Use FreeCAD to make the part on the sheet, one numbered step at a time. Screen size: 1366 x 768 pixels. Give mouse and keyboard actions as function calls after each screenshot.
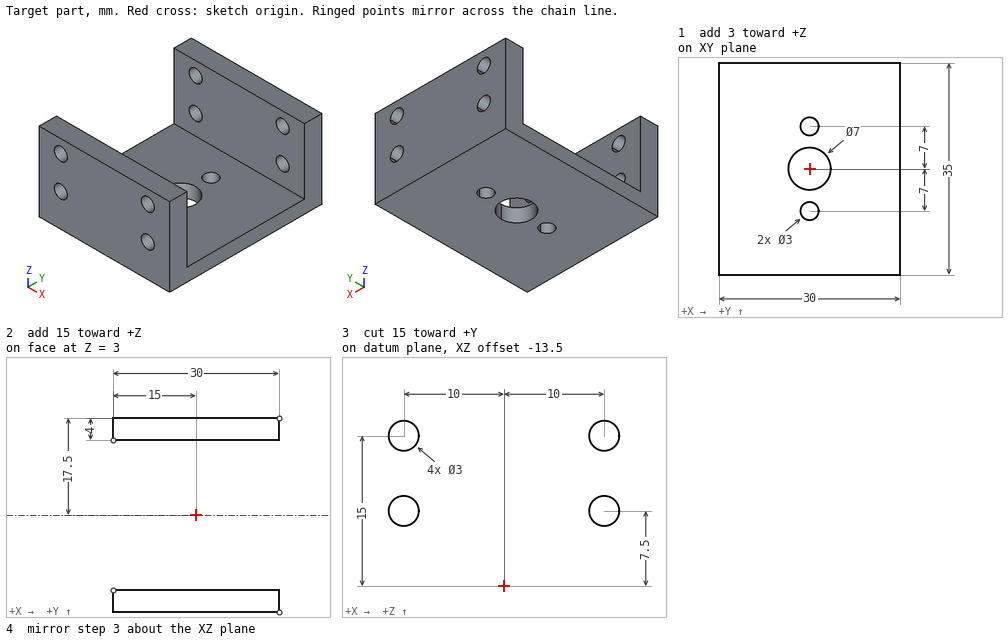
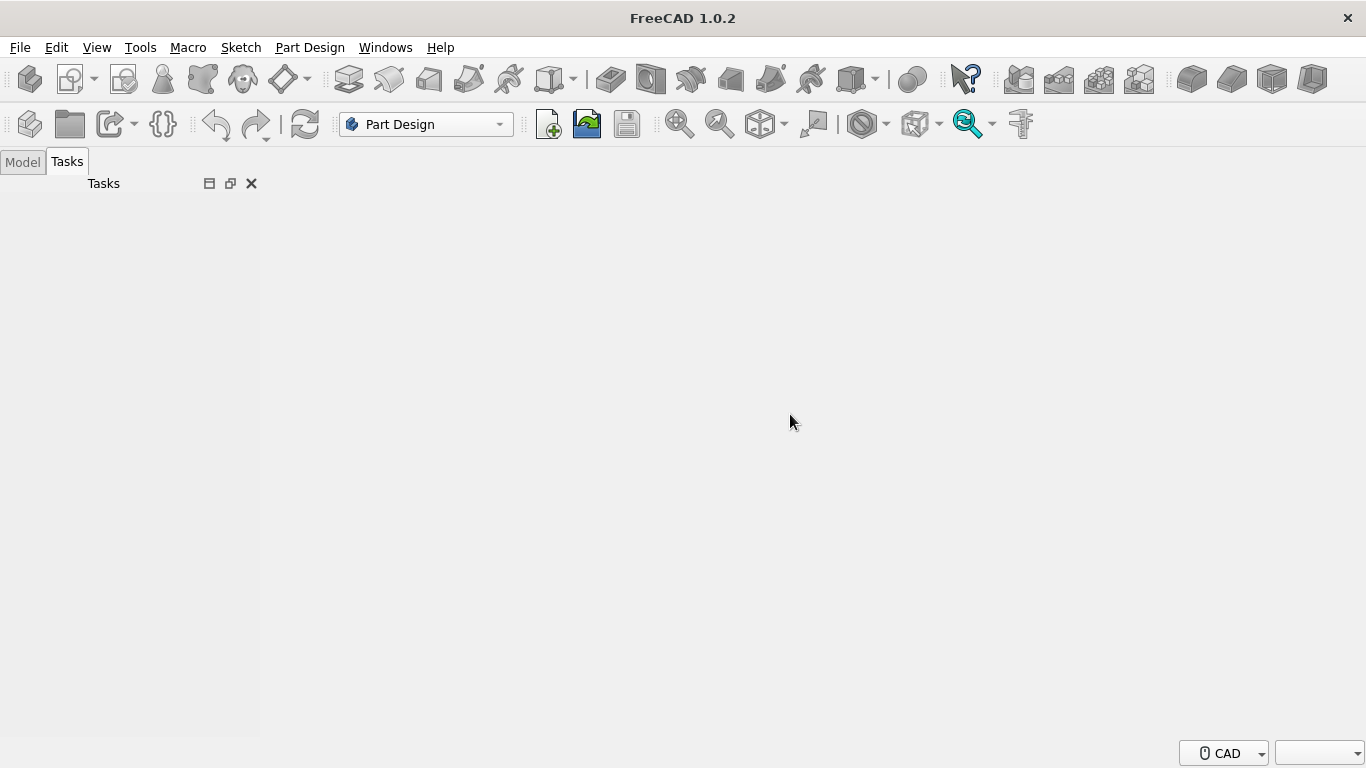
click(548, 124)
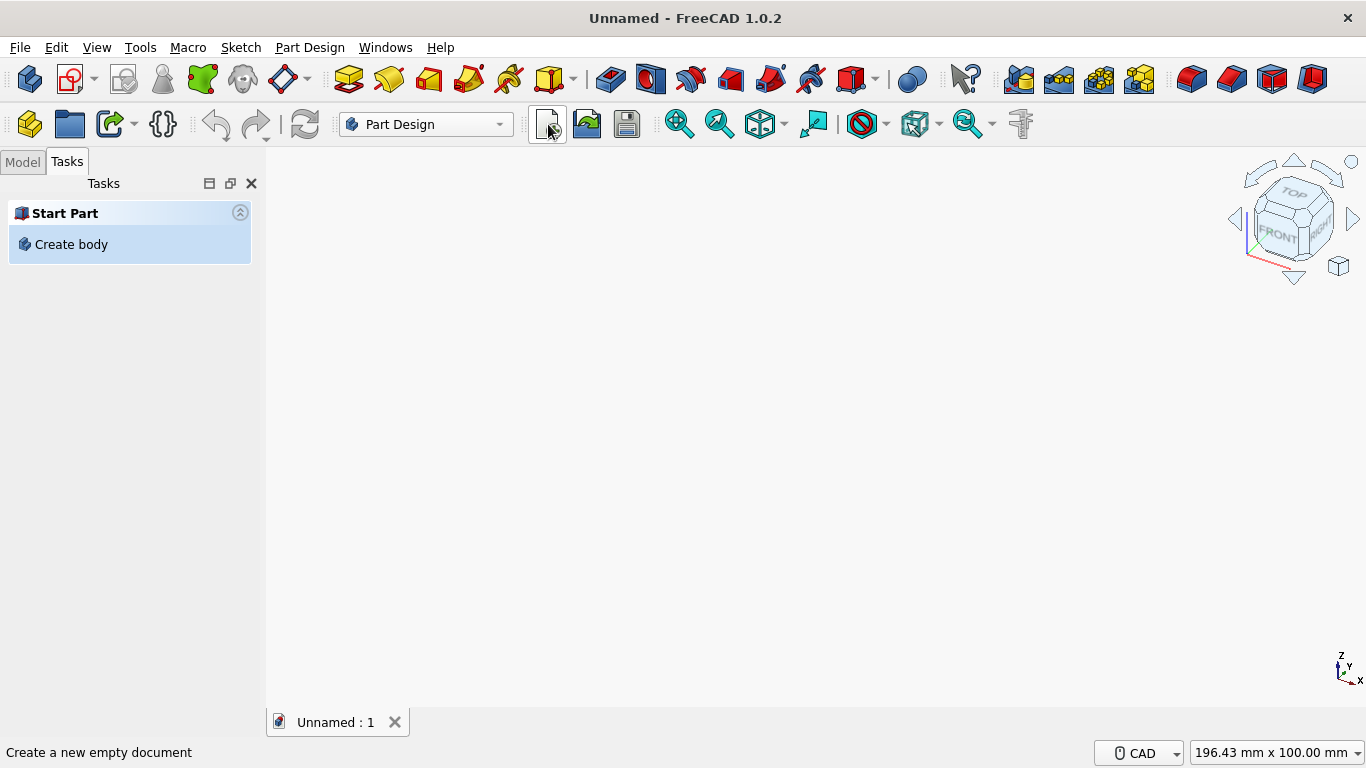
click(70, 80)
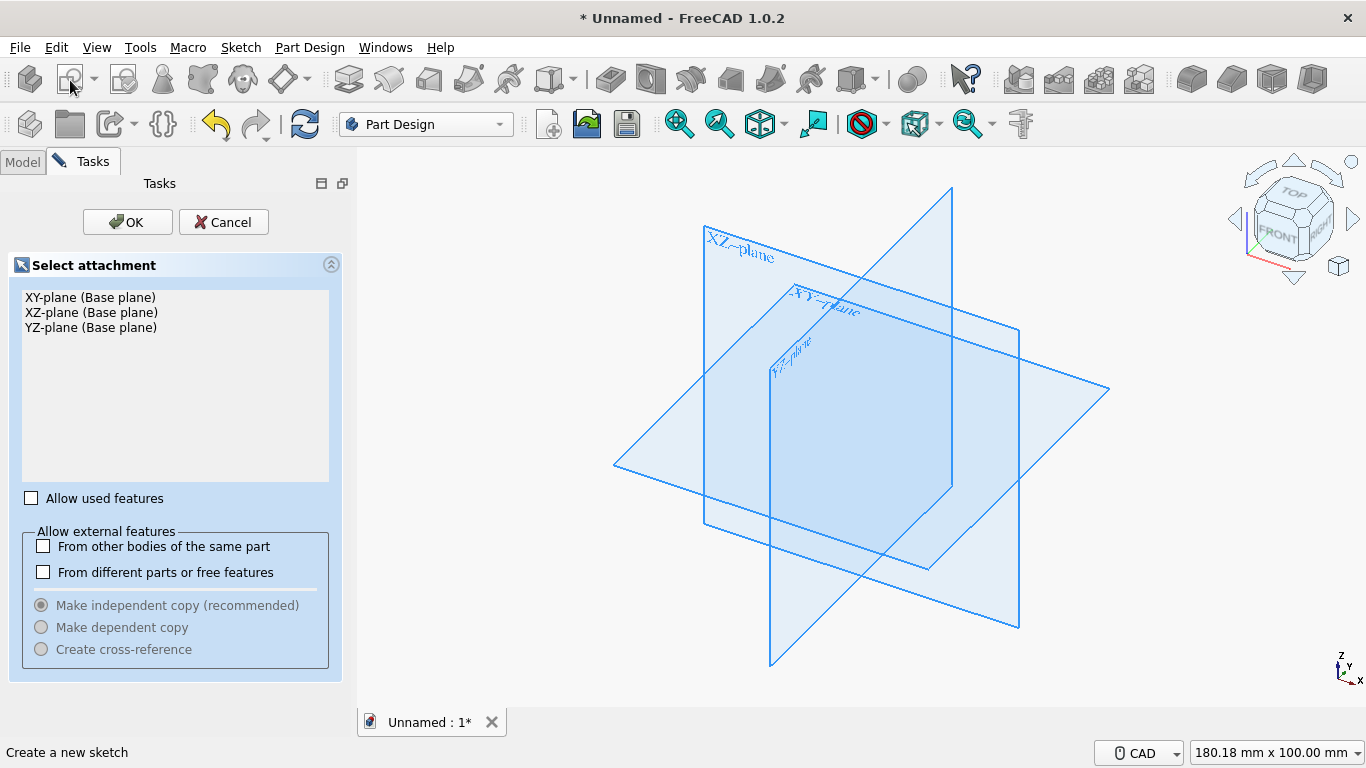
click(82, 298)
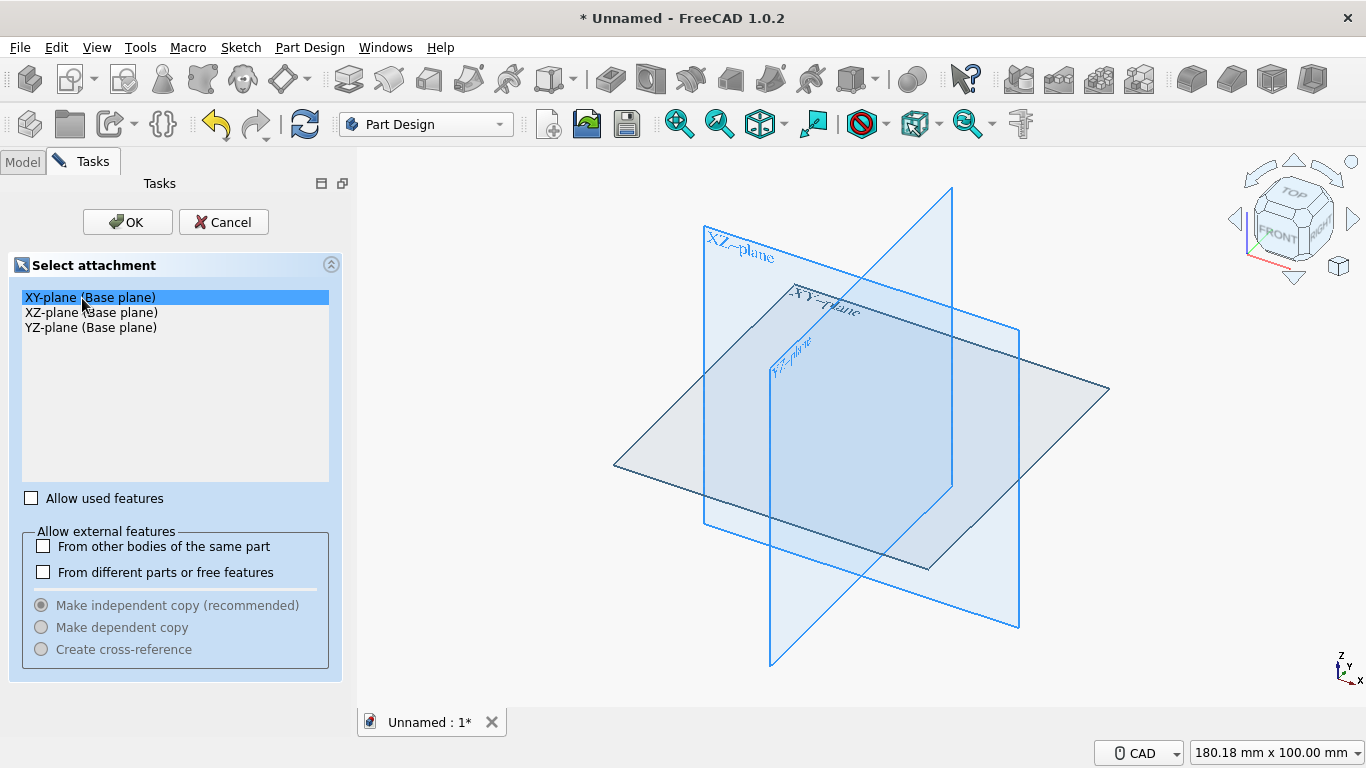
click(128, 222)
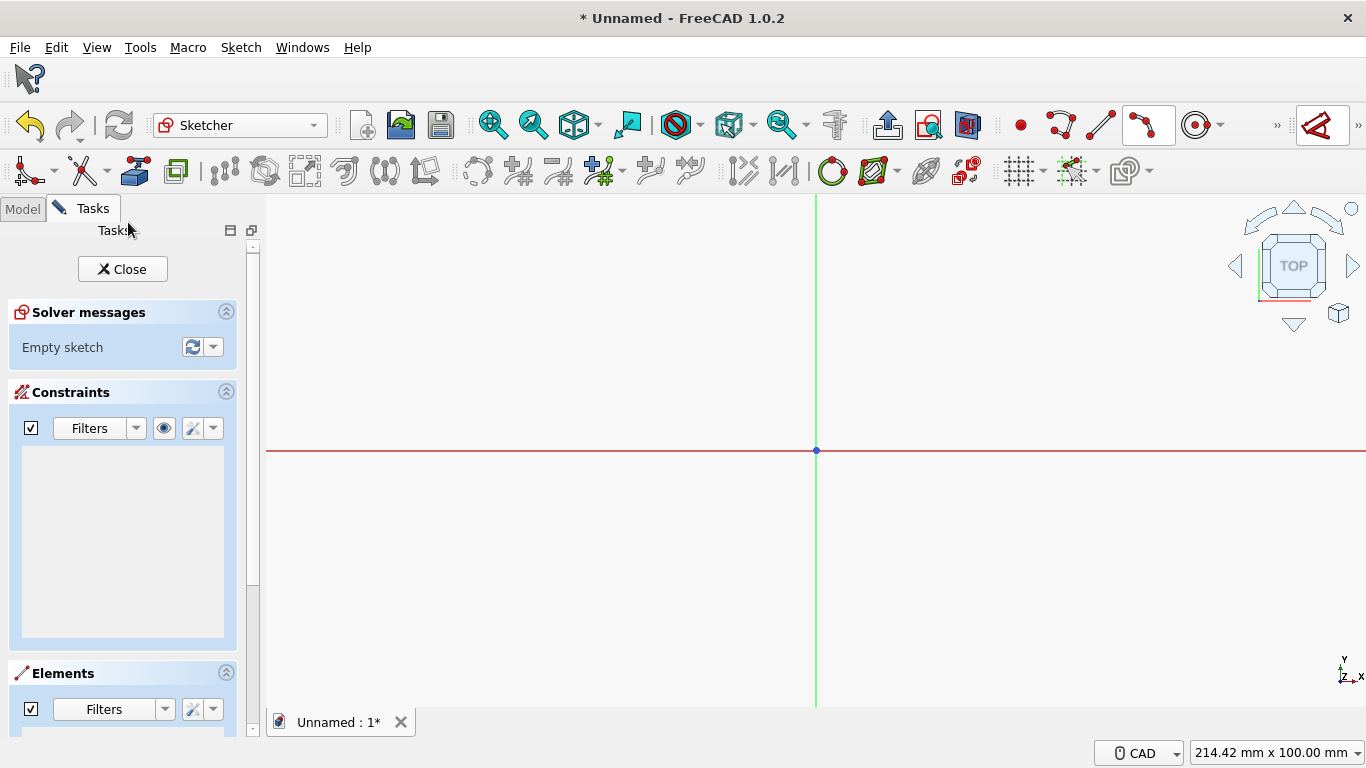
scroll(899, 450, up, 3)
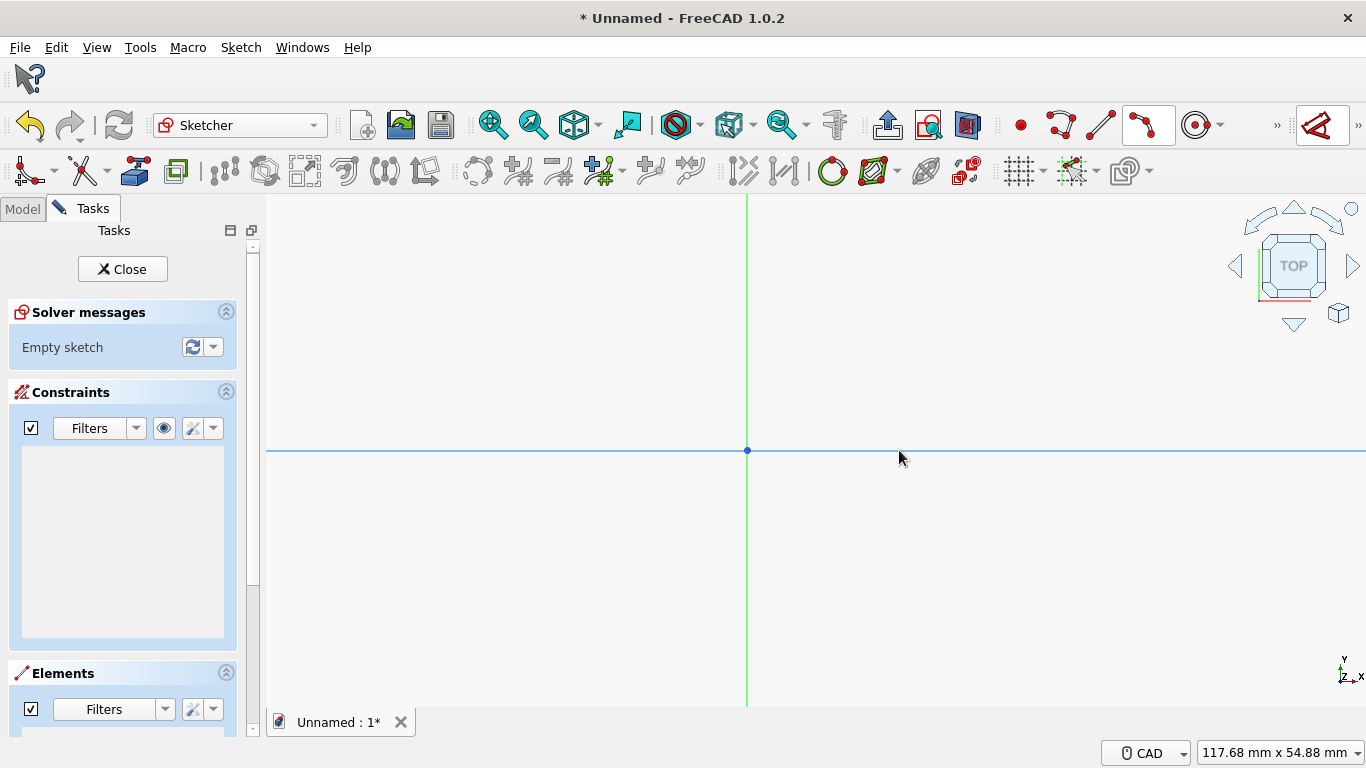
key(g)
key(v)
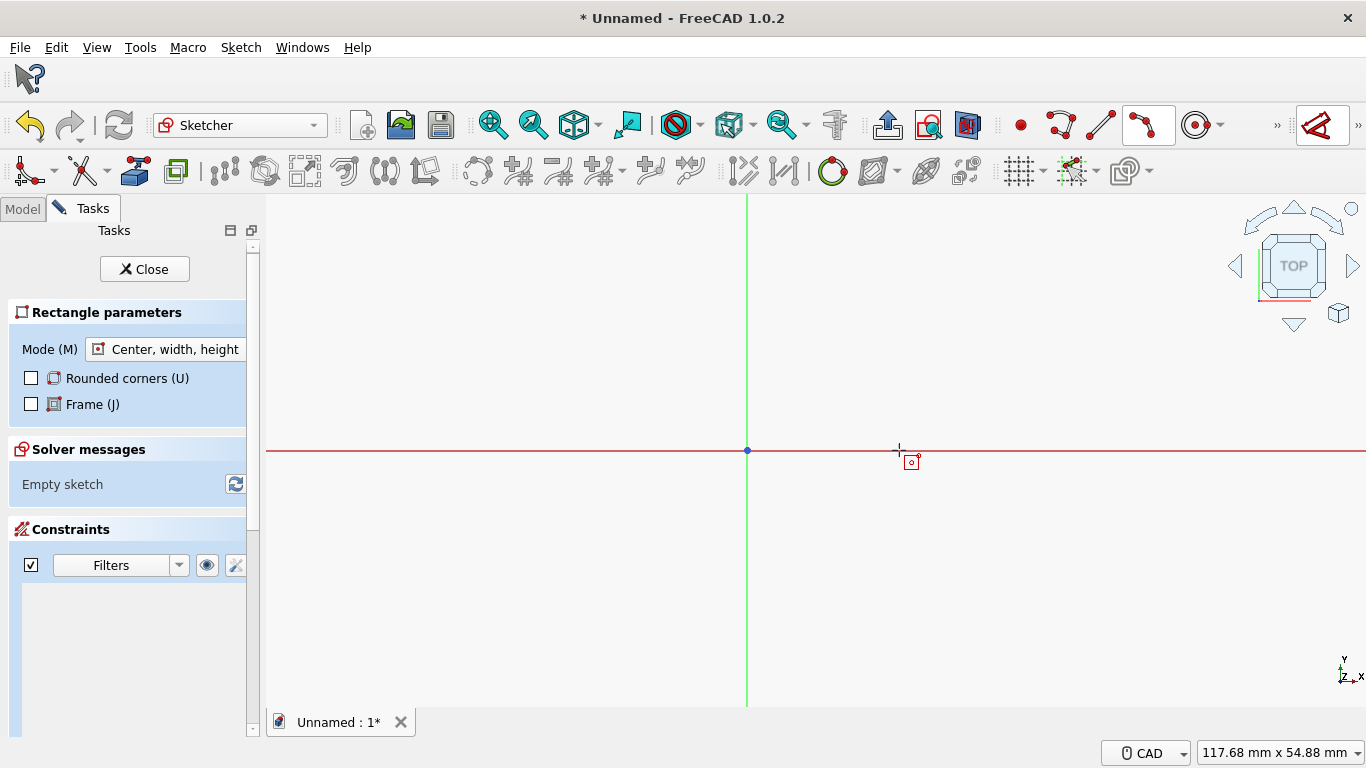
click(747, 450)
click(888, 287)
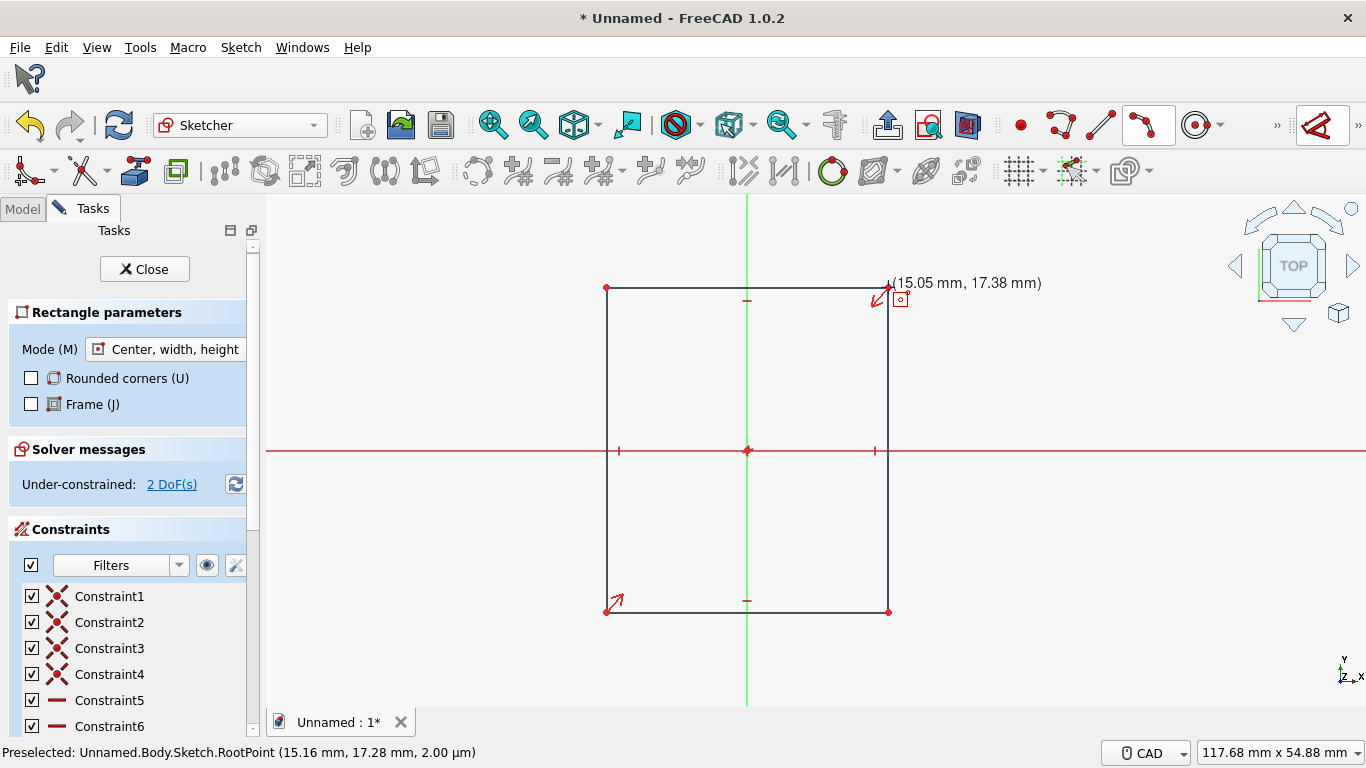
click(1196, 126)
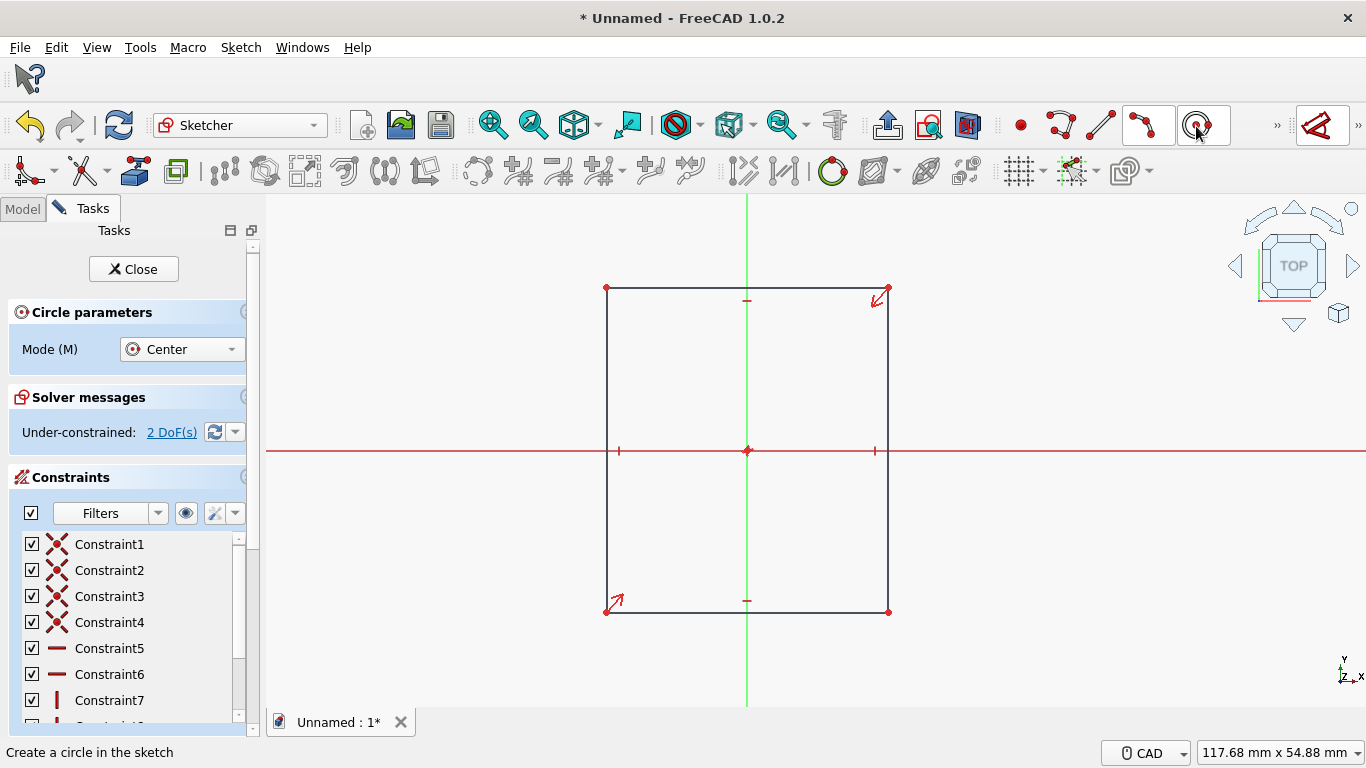
scroll(747, 516, up, 3)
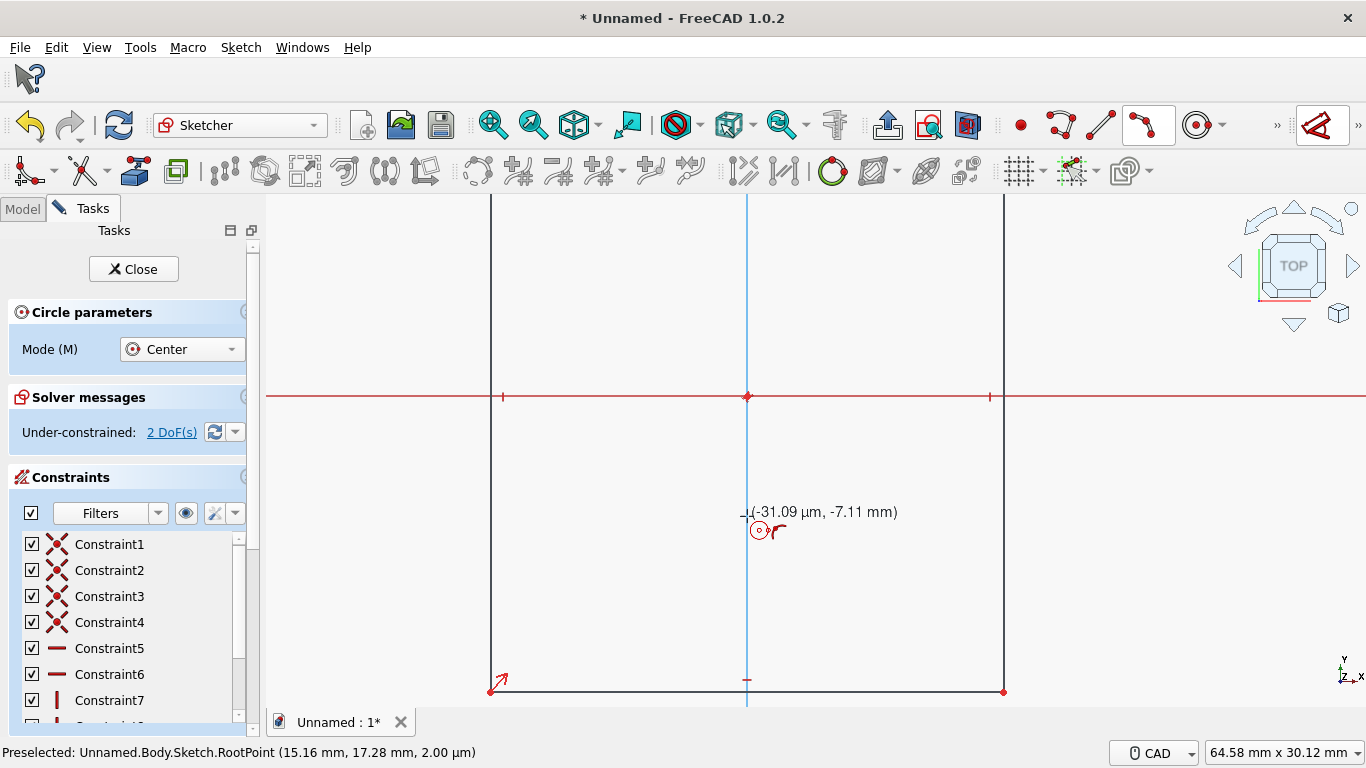
click(747, 515)
click(765, 497)